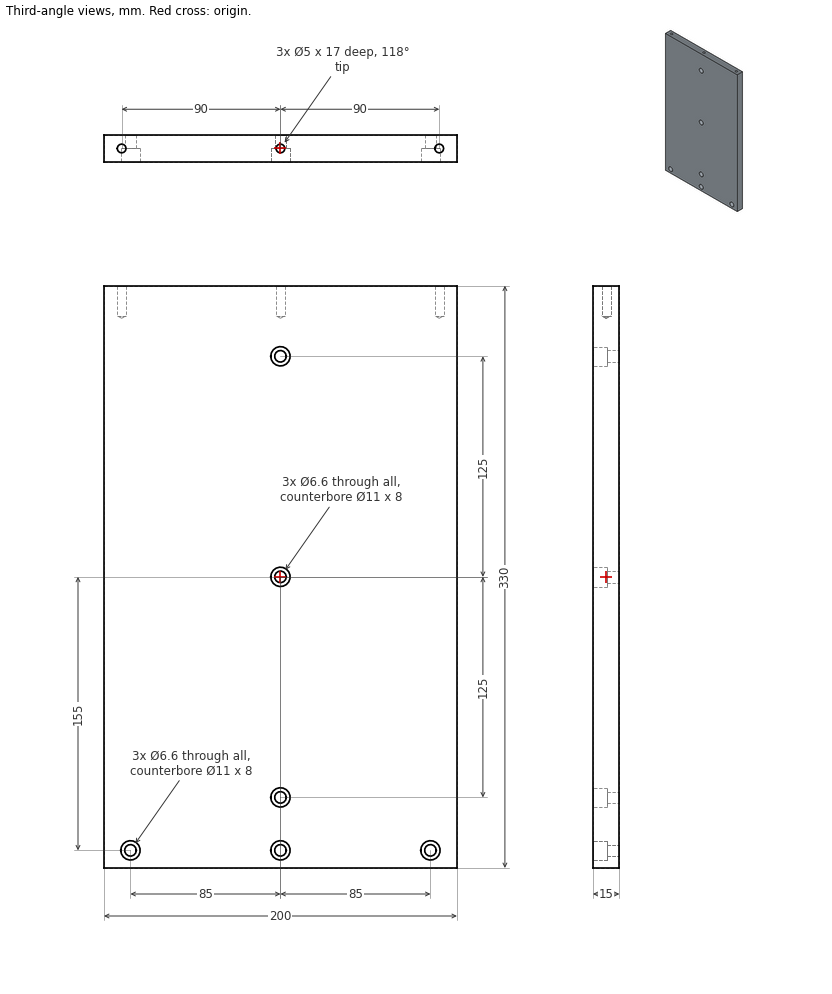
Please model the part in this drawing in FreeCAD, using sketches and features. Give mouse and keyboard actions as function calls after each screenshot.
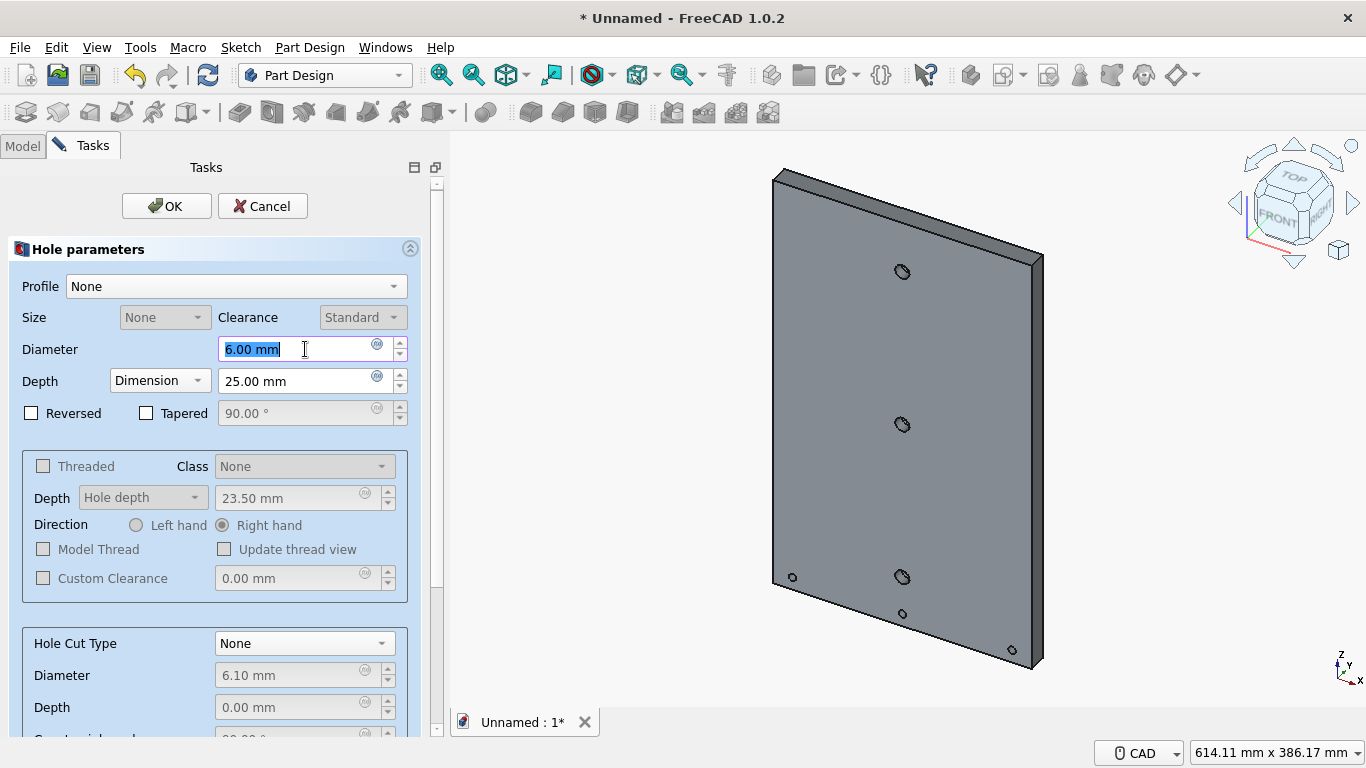
text(6.6)
key(Tab)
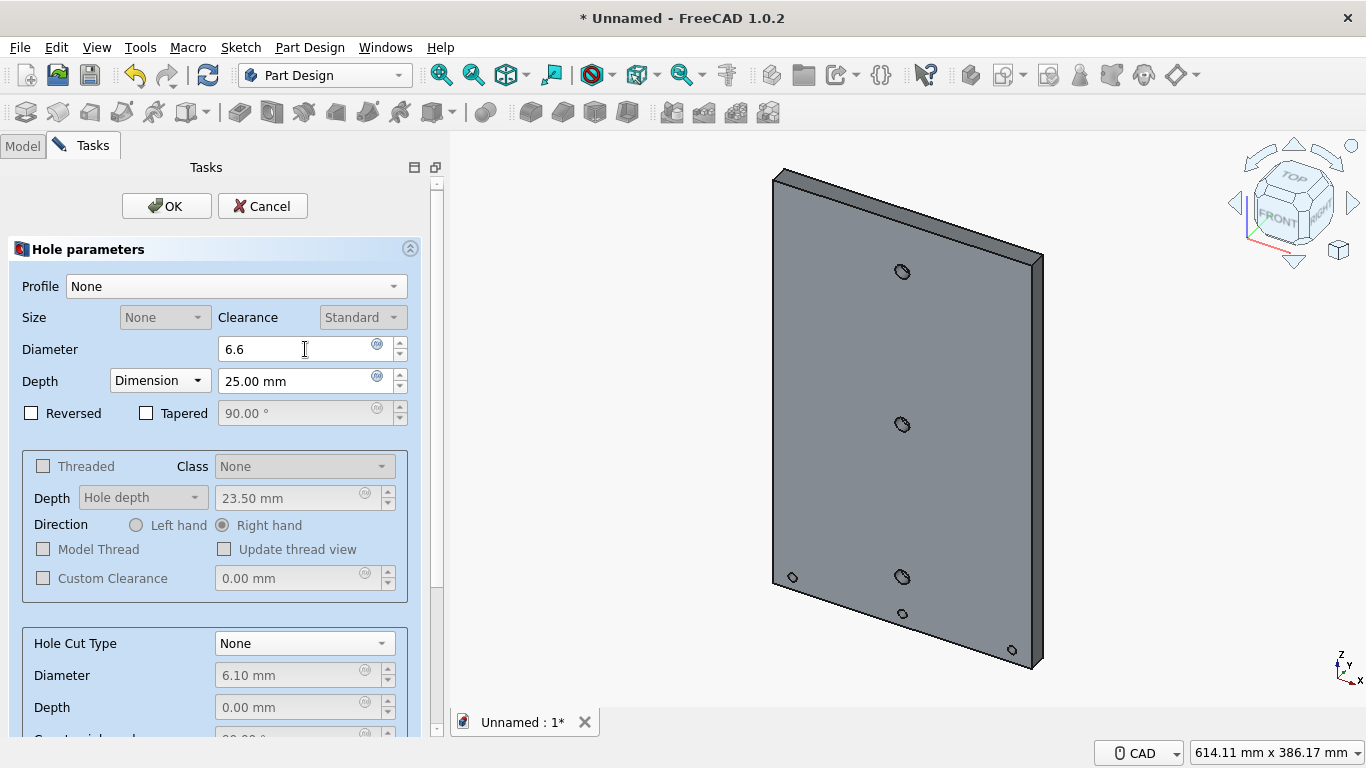
click(161, 380)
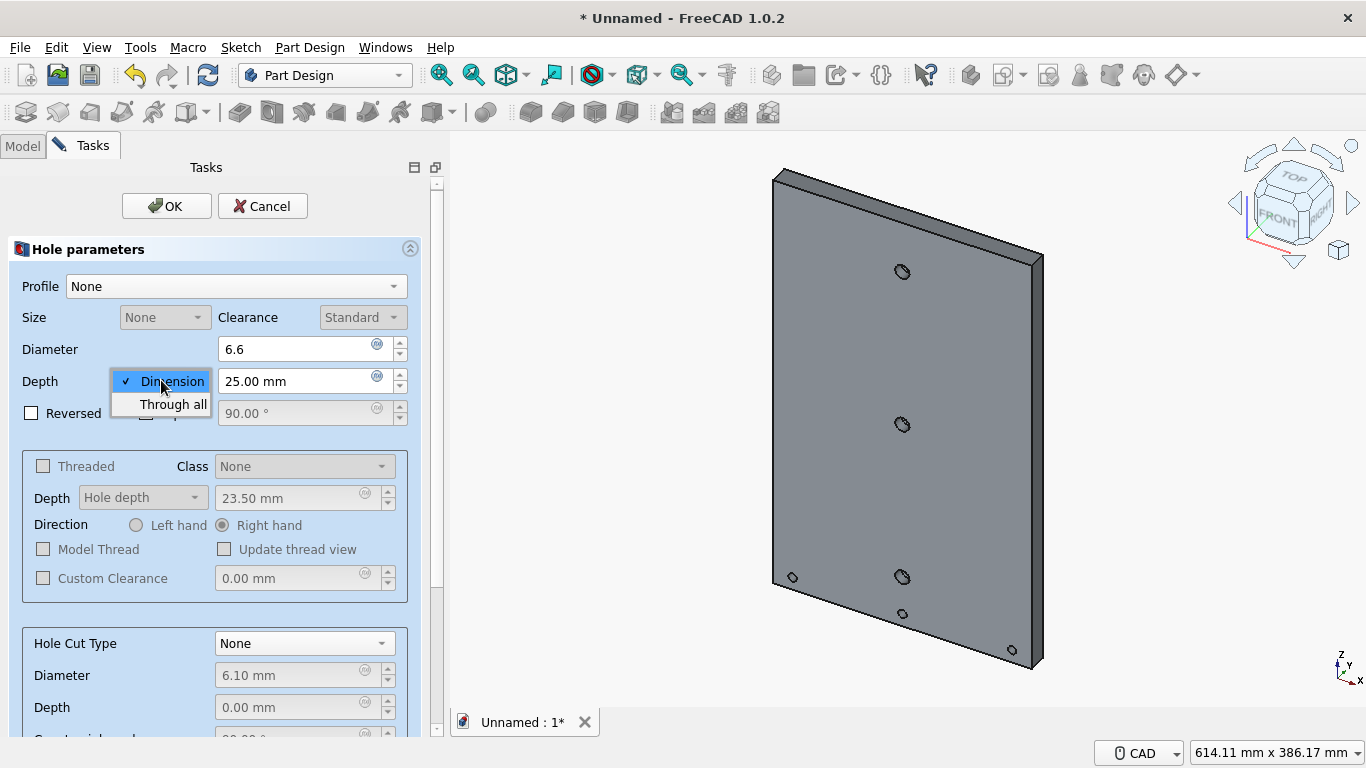
click(160, 404)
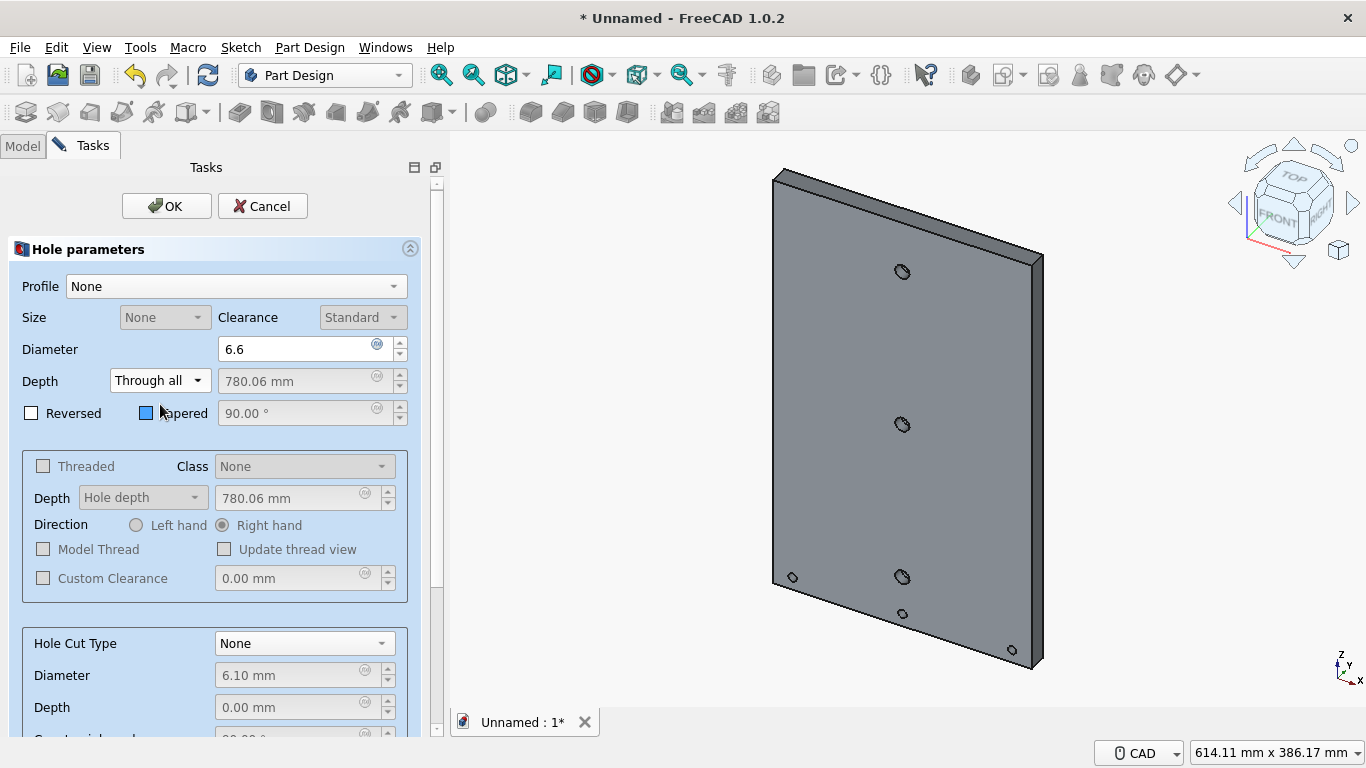
click(306, 644)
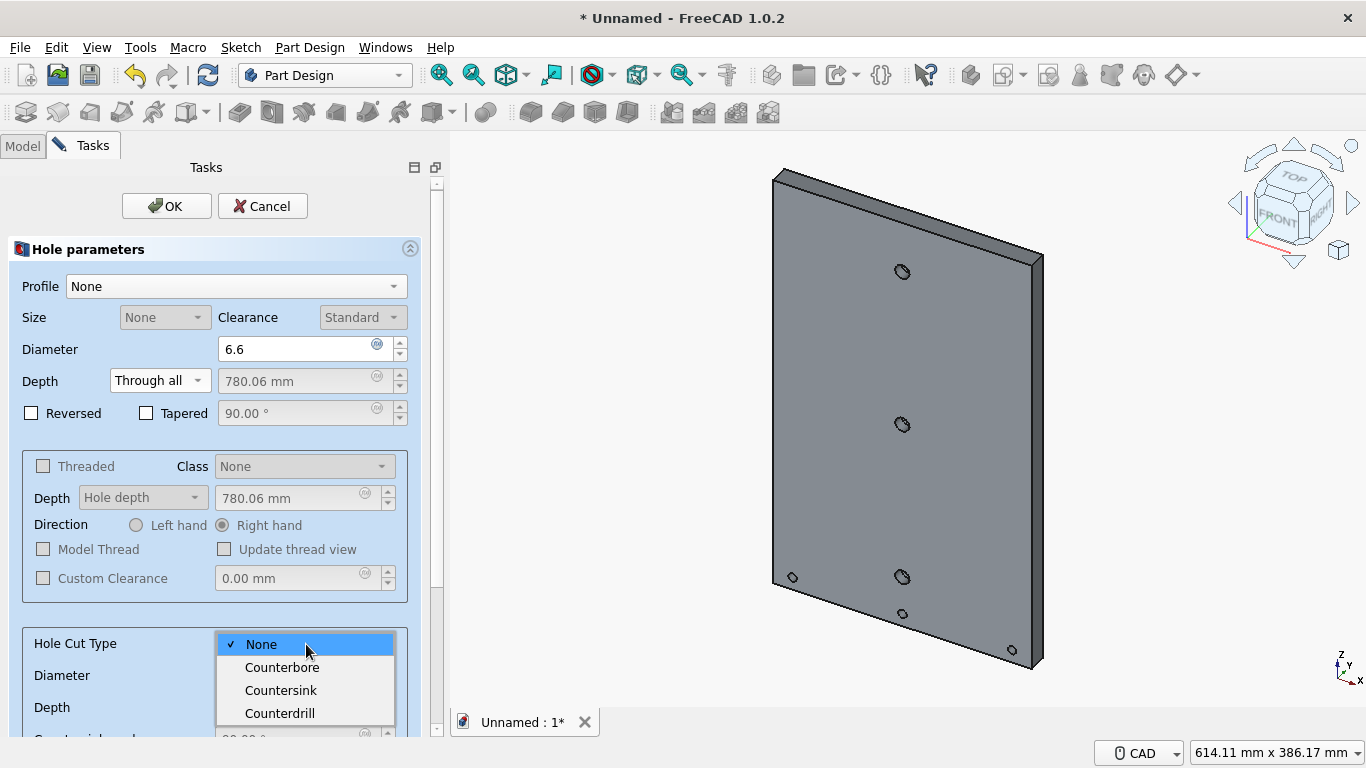
click(304, 668)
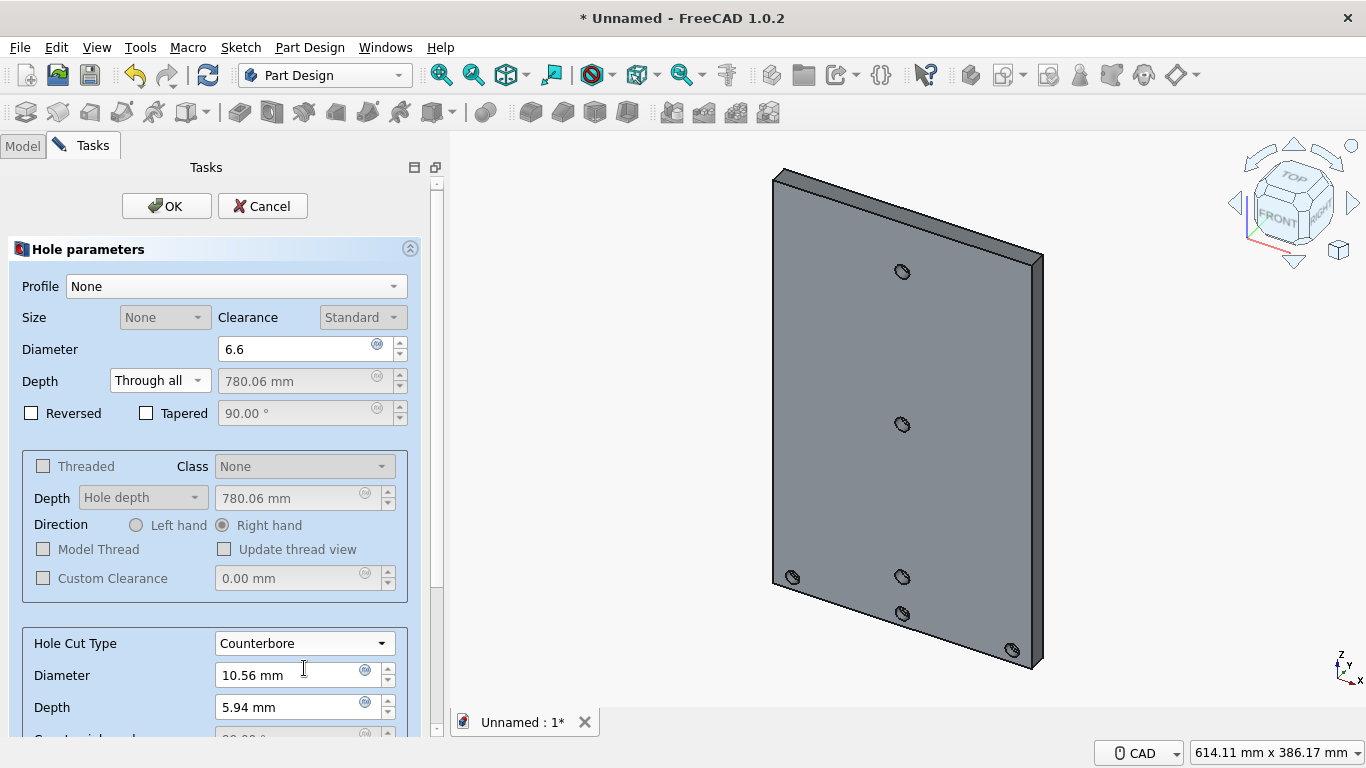
triple_click(298, 675)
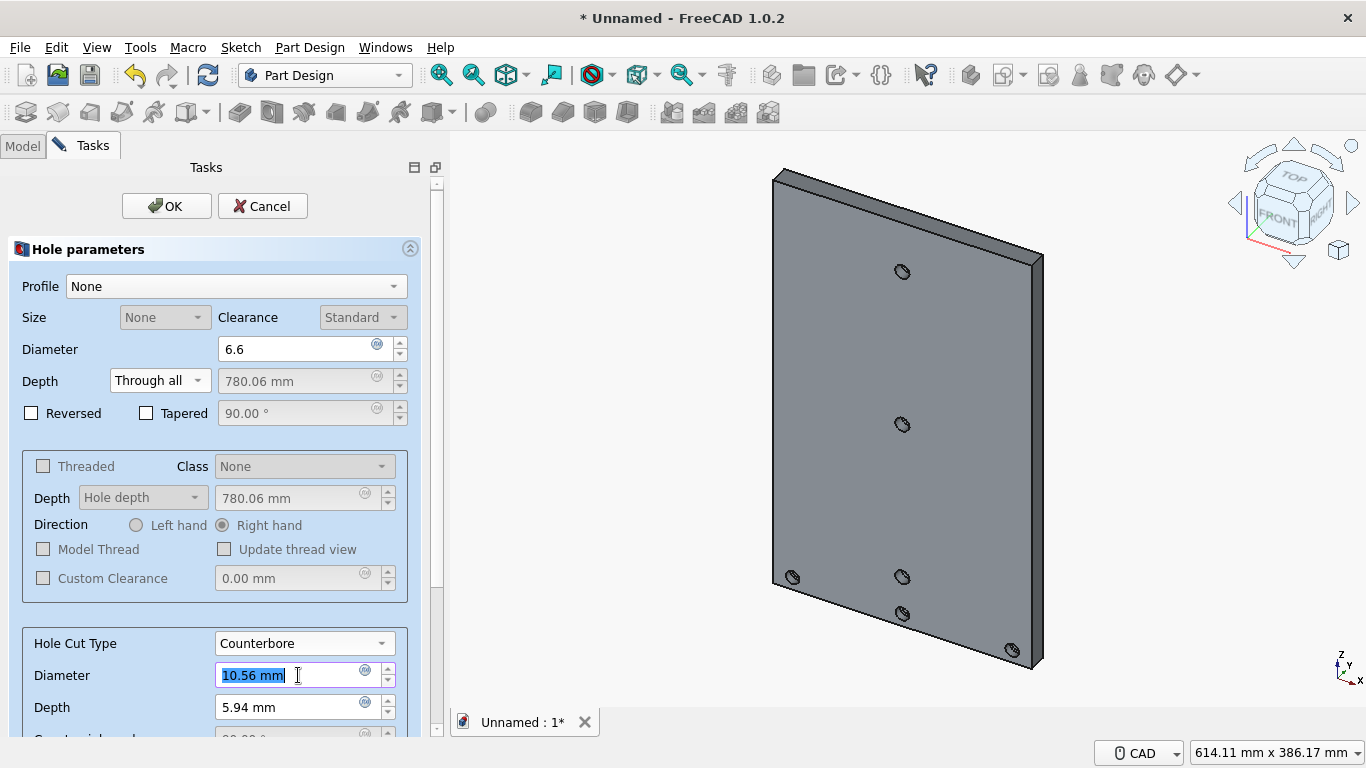
text(11)
key(Tab)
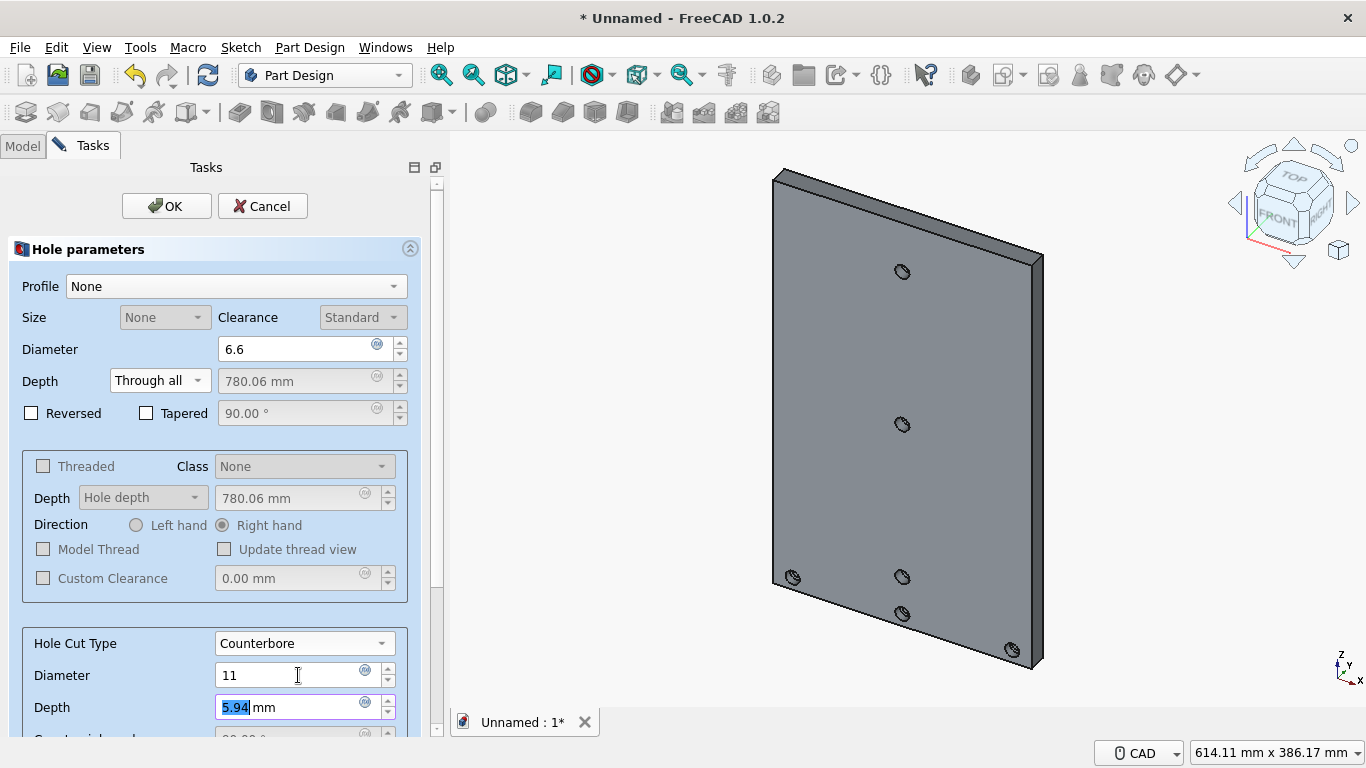
text(8)
key(Tab)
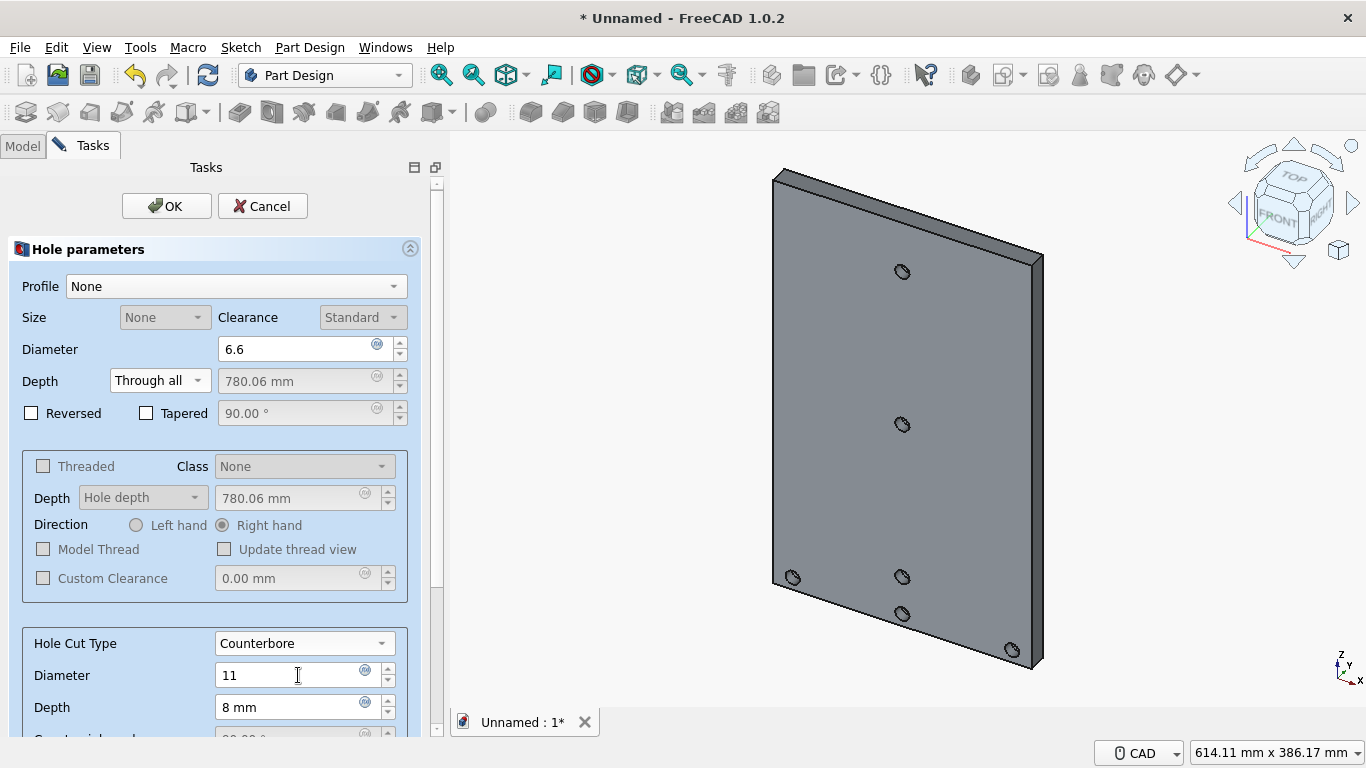
click(167, 206)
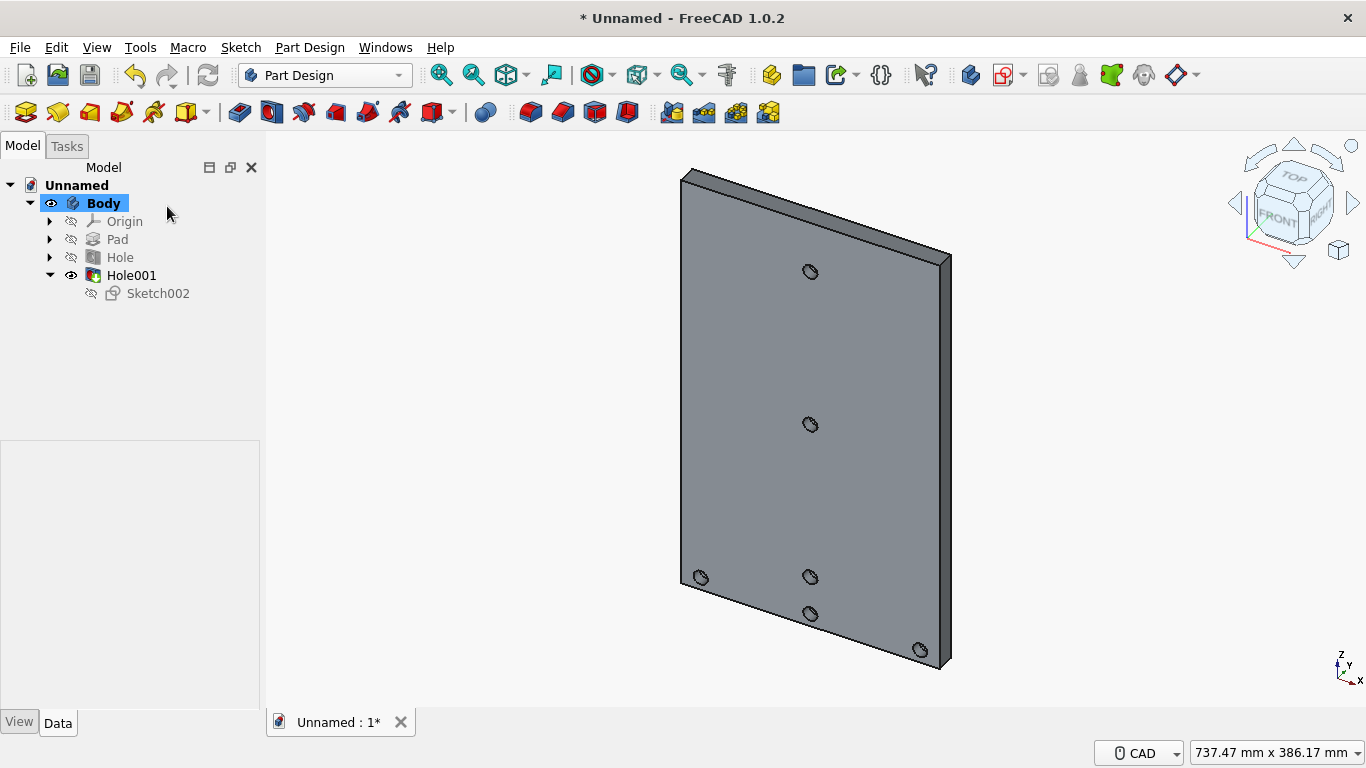
click(928, 251)